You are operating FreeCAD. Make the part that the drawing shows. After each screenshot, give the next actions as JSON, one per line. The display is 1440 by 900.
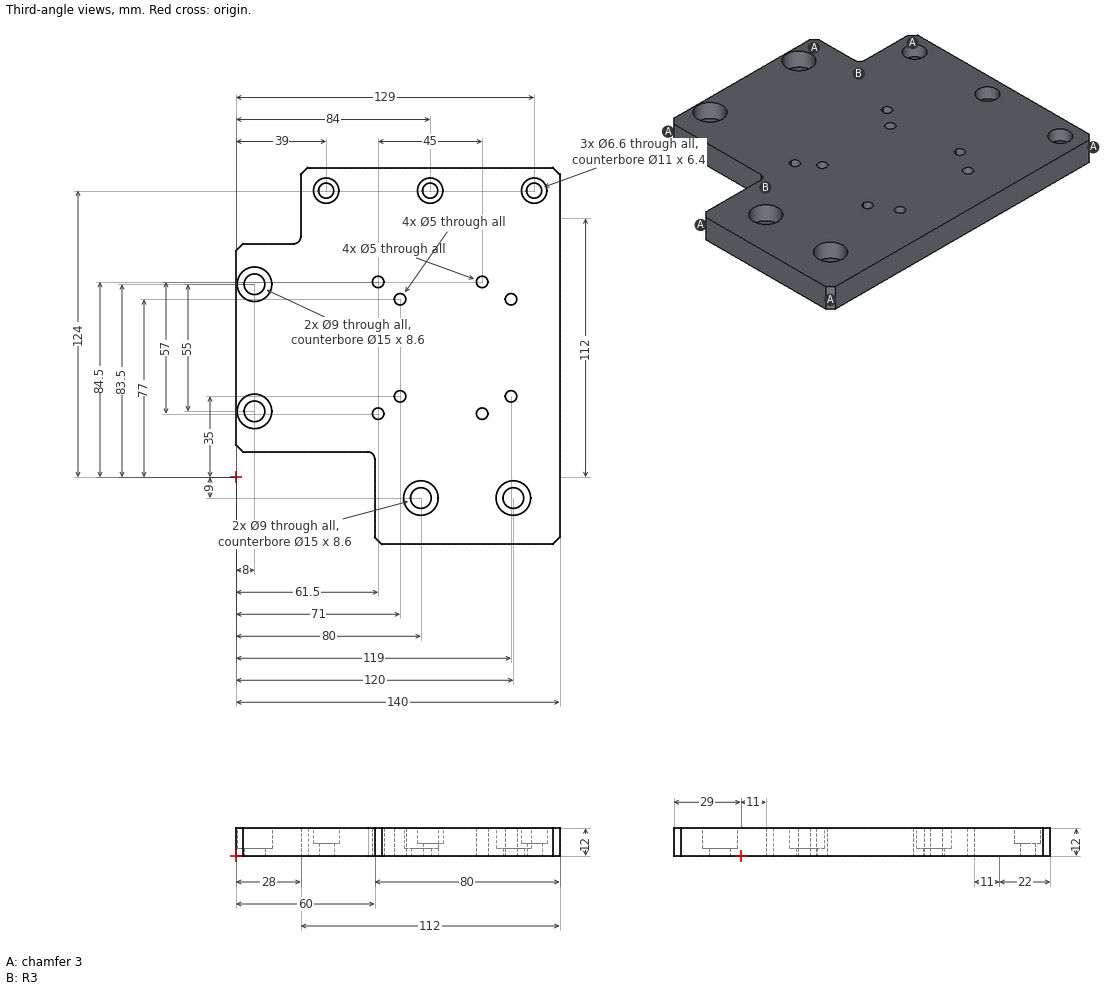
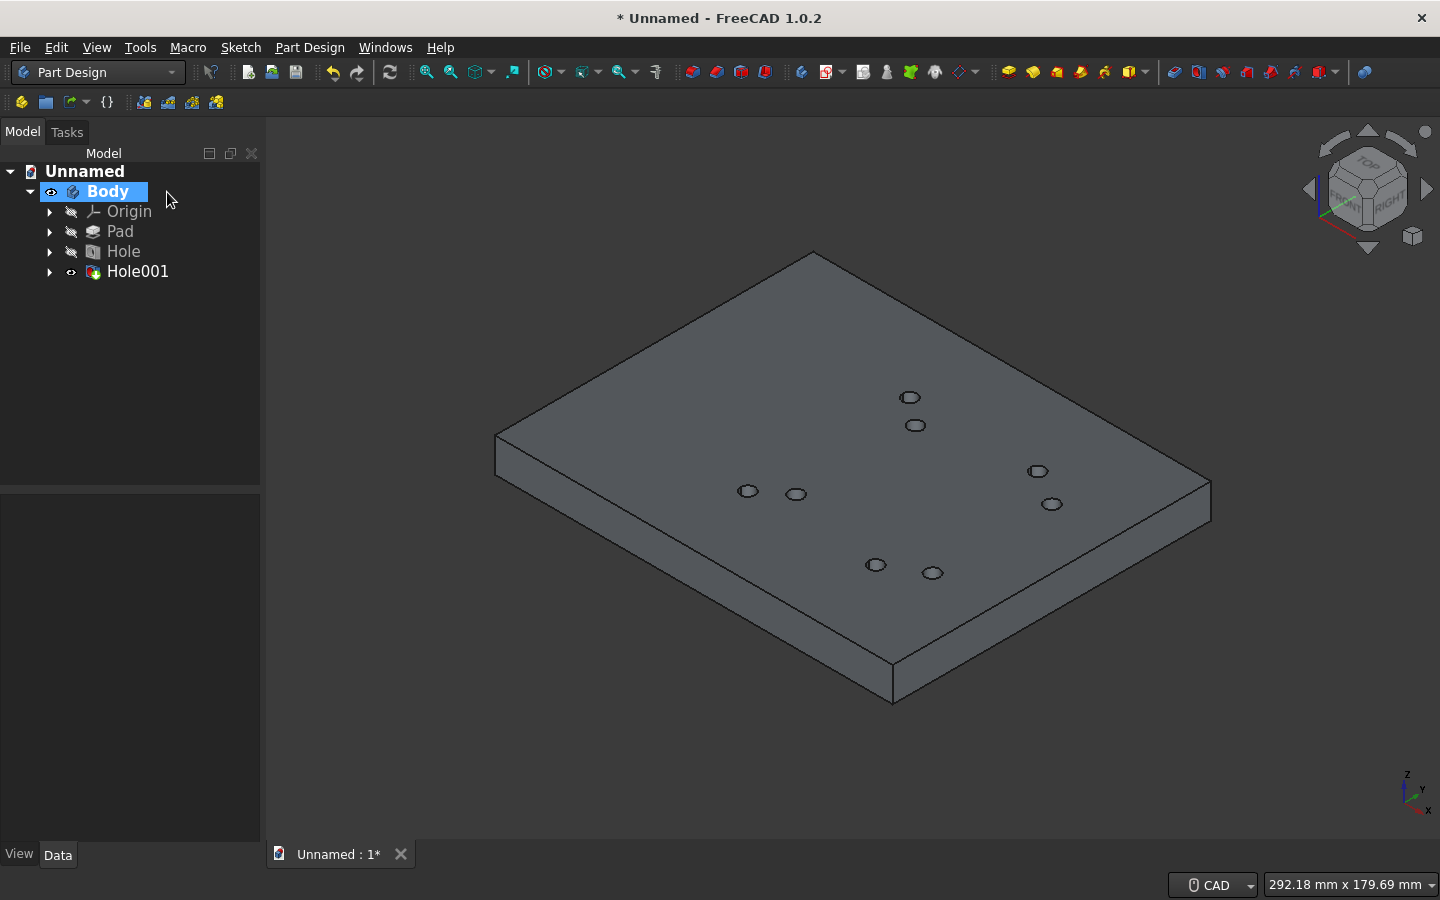
{"action": "key", "text": "4"}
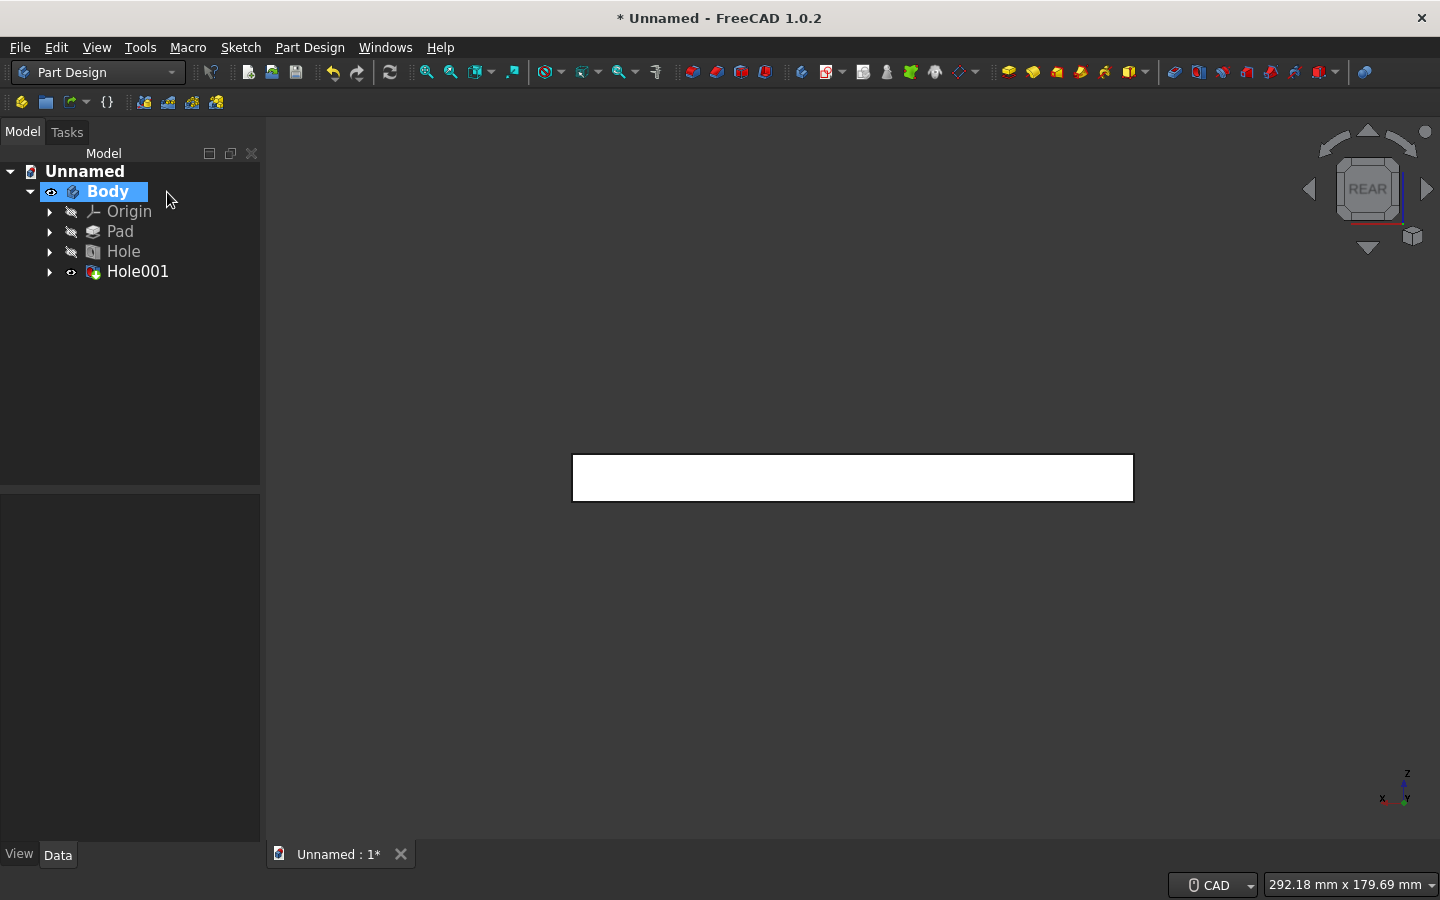
{"action": "left_click", "coordinate": [612, 477]}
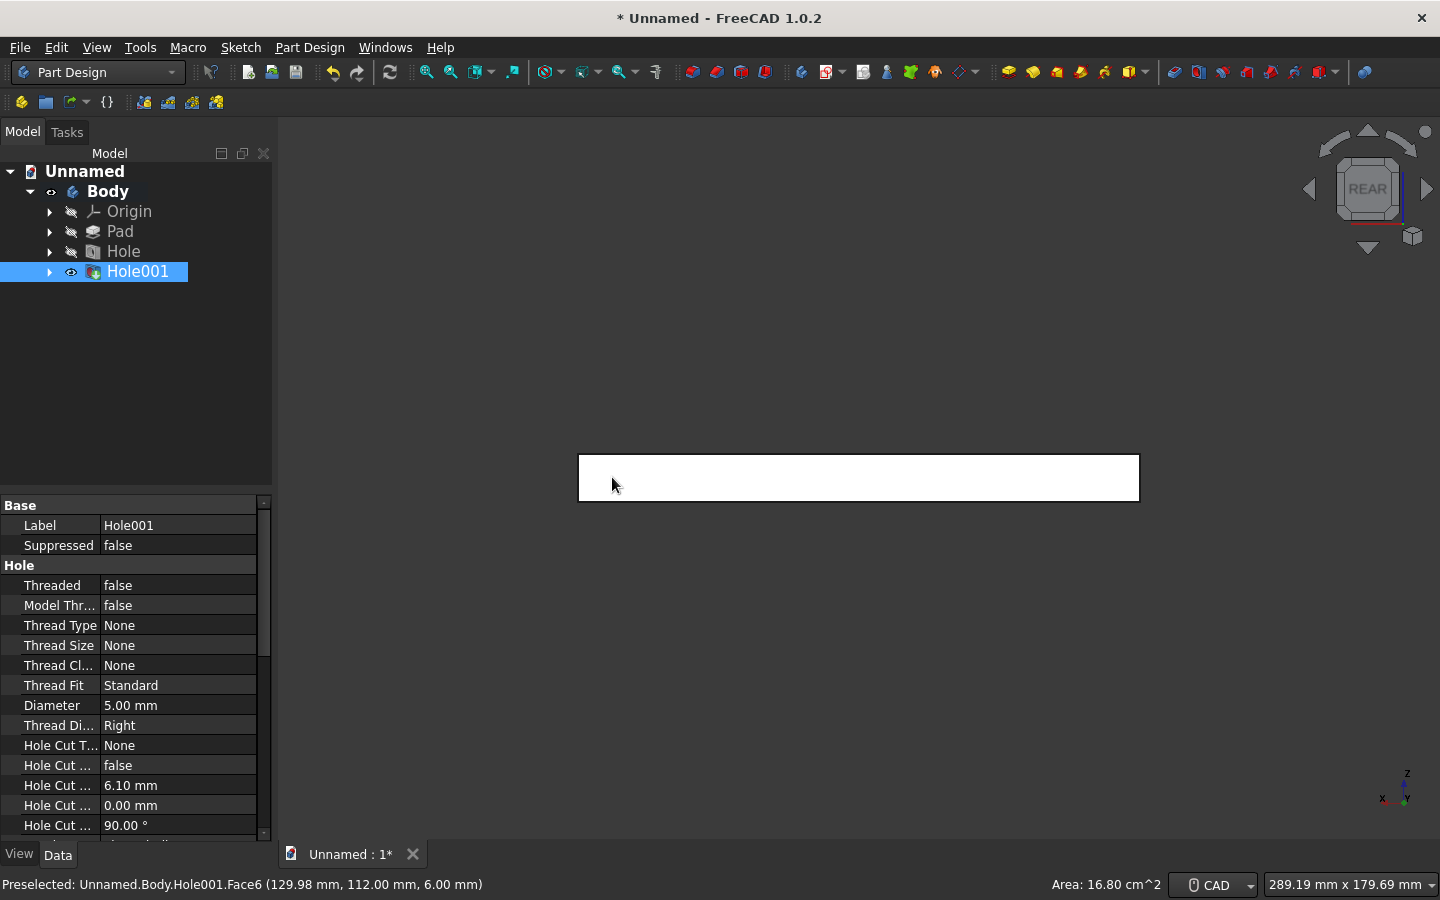
{"action": "left_click", "coordinate": [826, 72]}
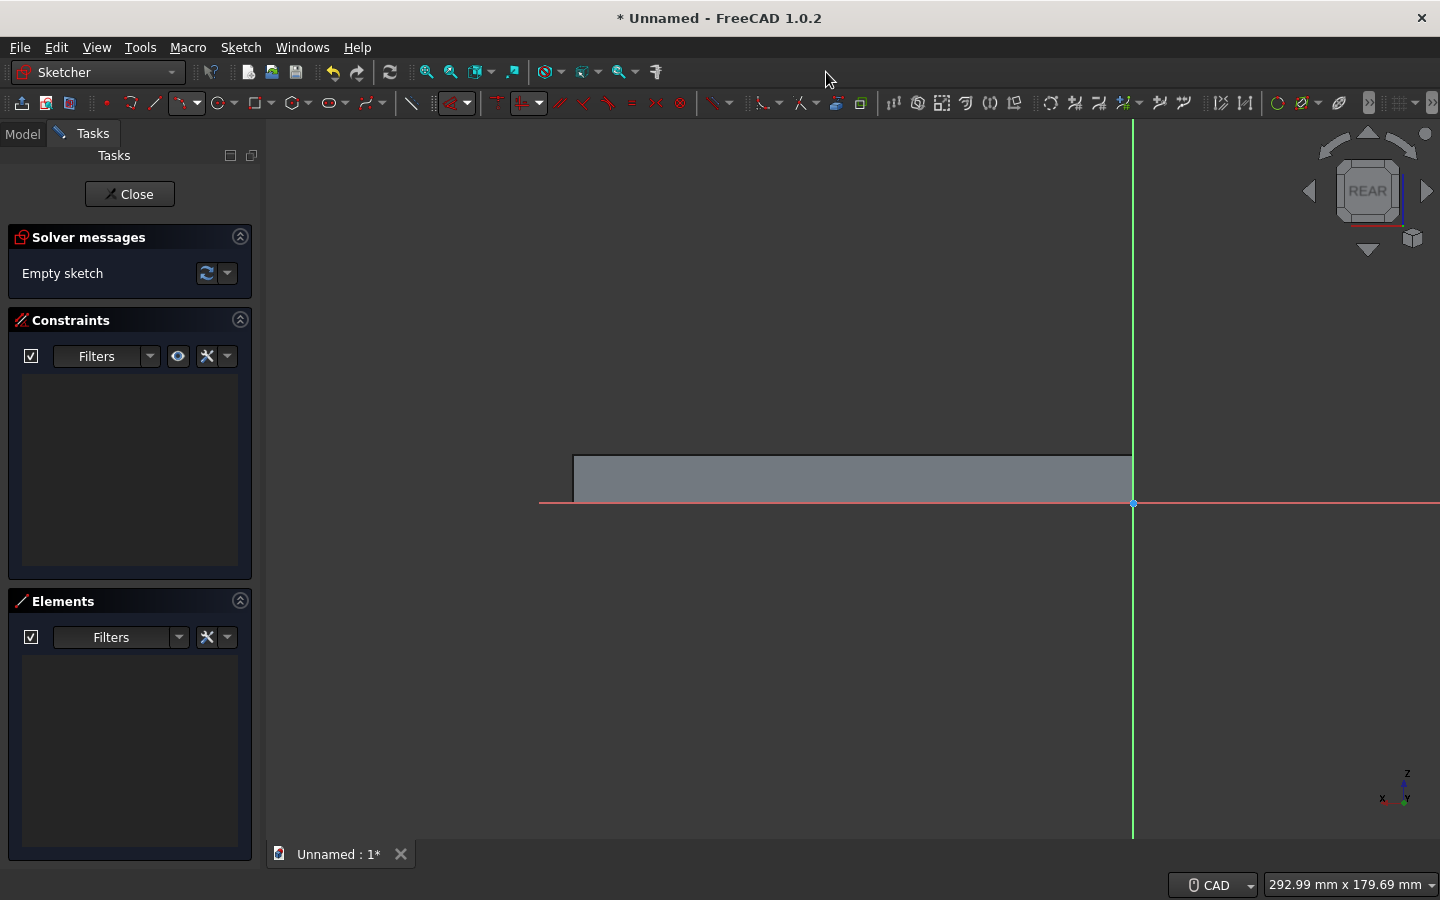
{"action": "key", "text": "g r"}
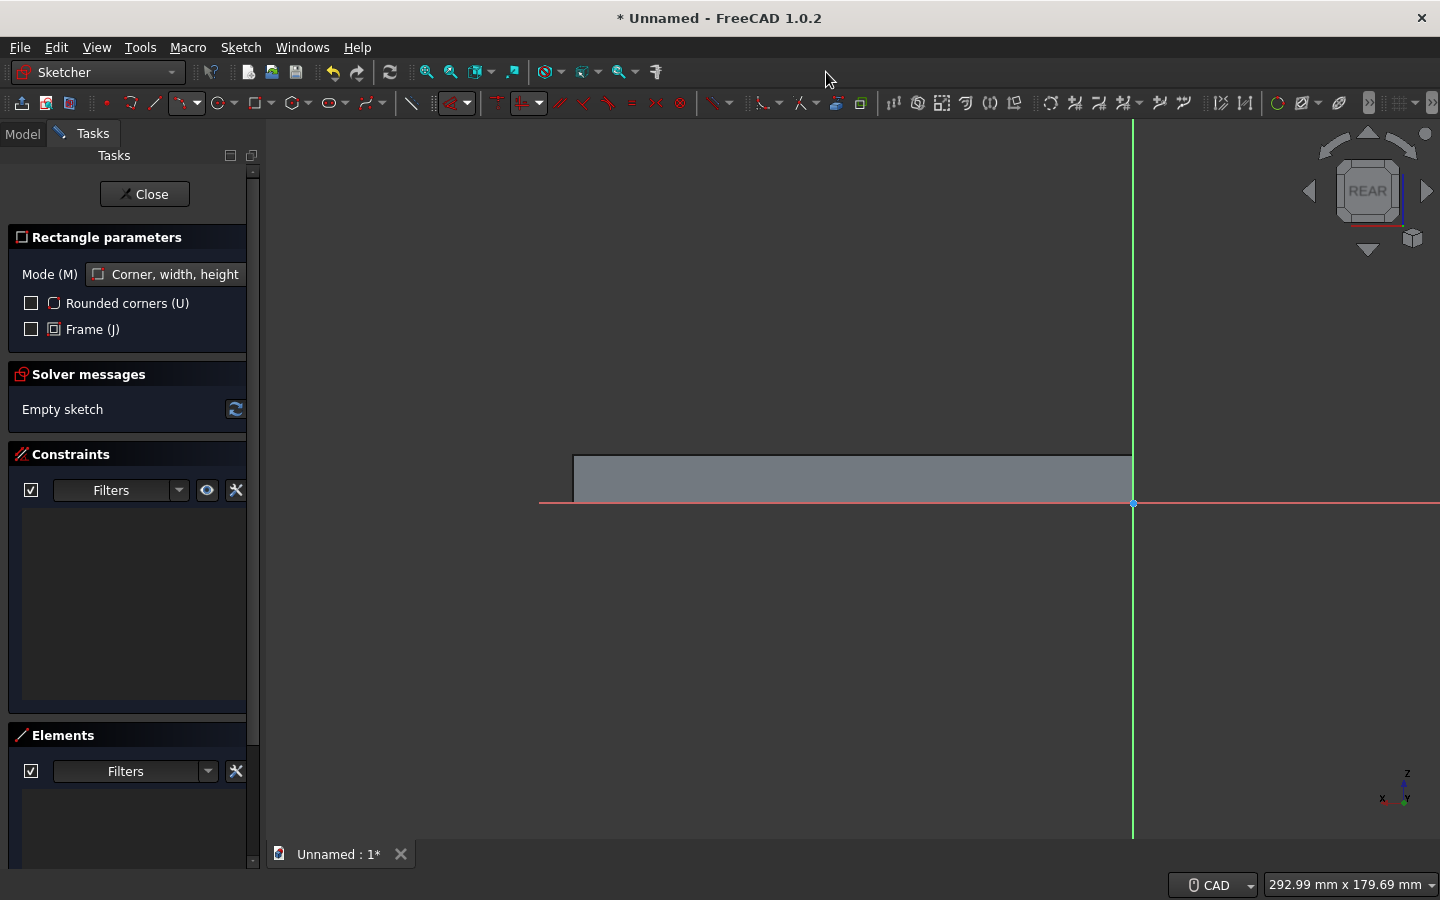
{"action": "left_click", "coordinate": [573, 455]}
{"action": "left_click", "coordinate": [1021, 503]}
{"action": "key", "text": "Escape"}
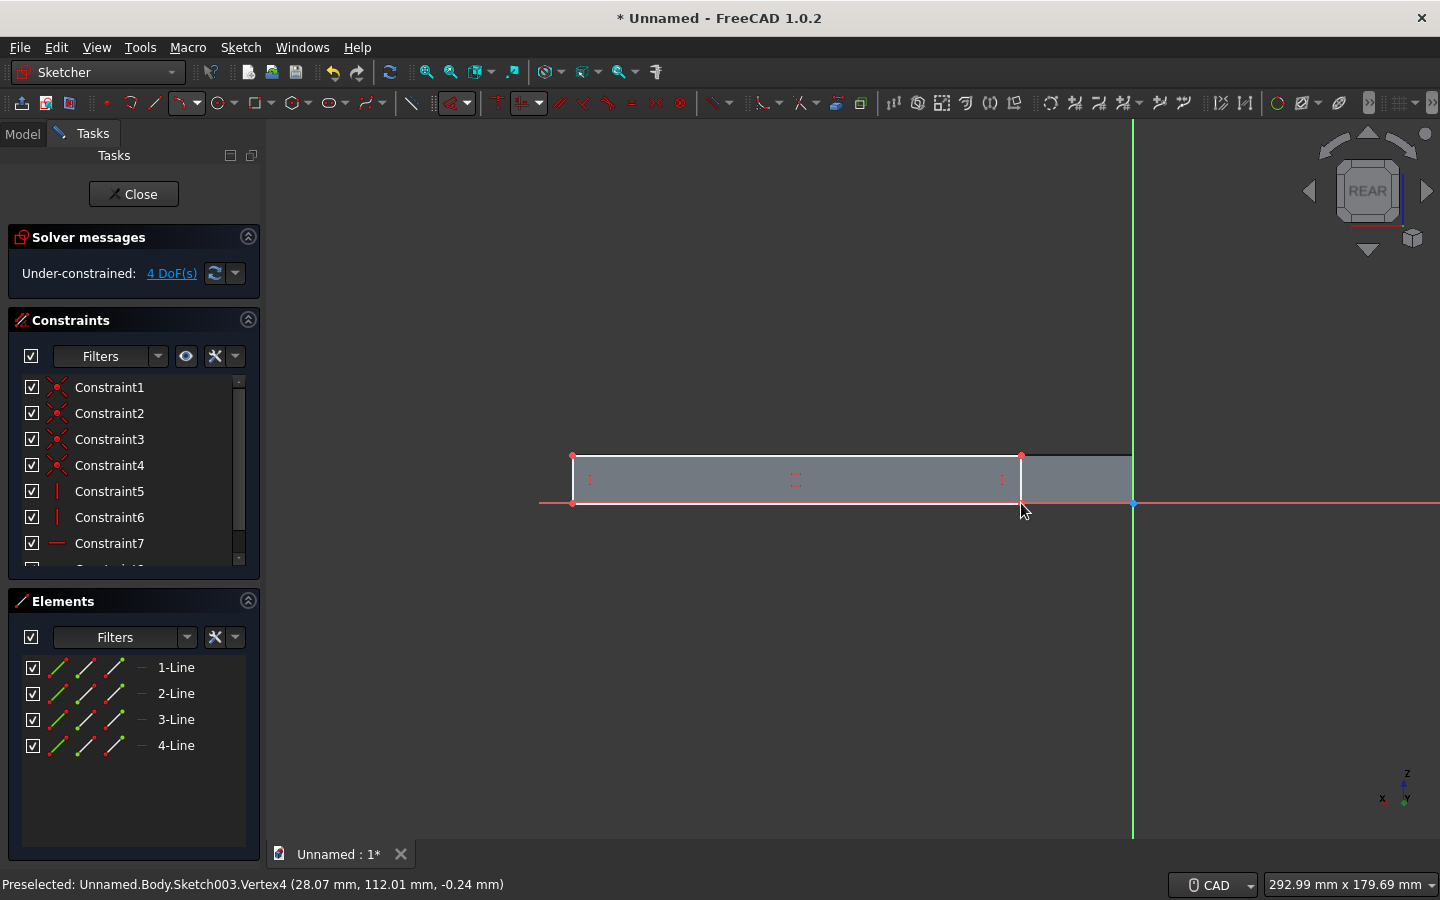
{"action": "left_click", "coordinate": [573, 504]}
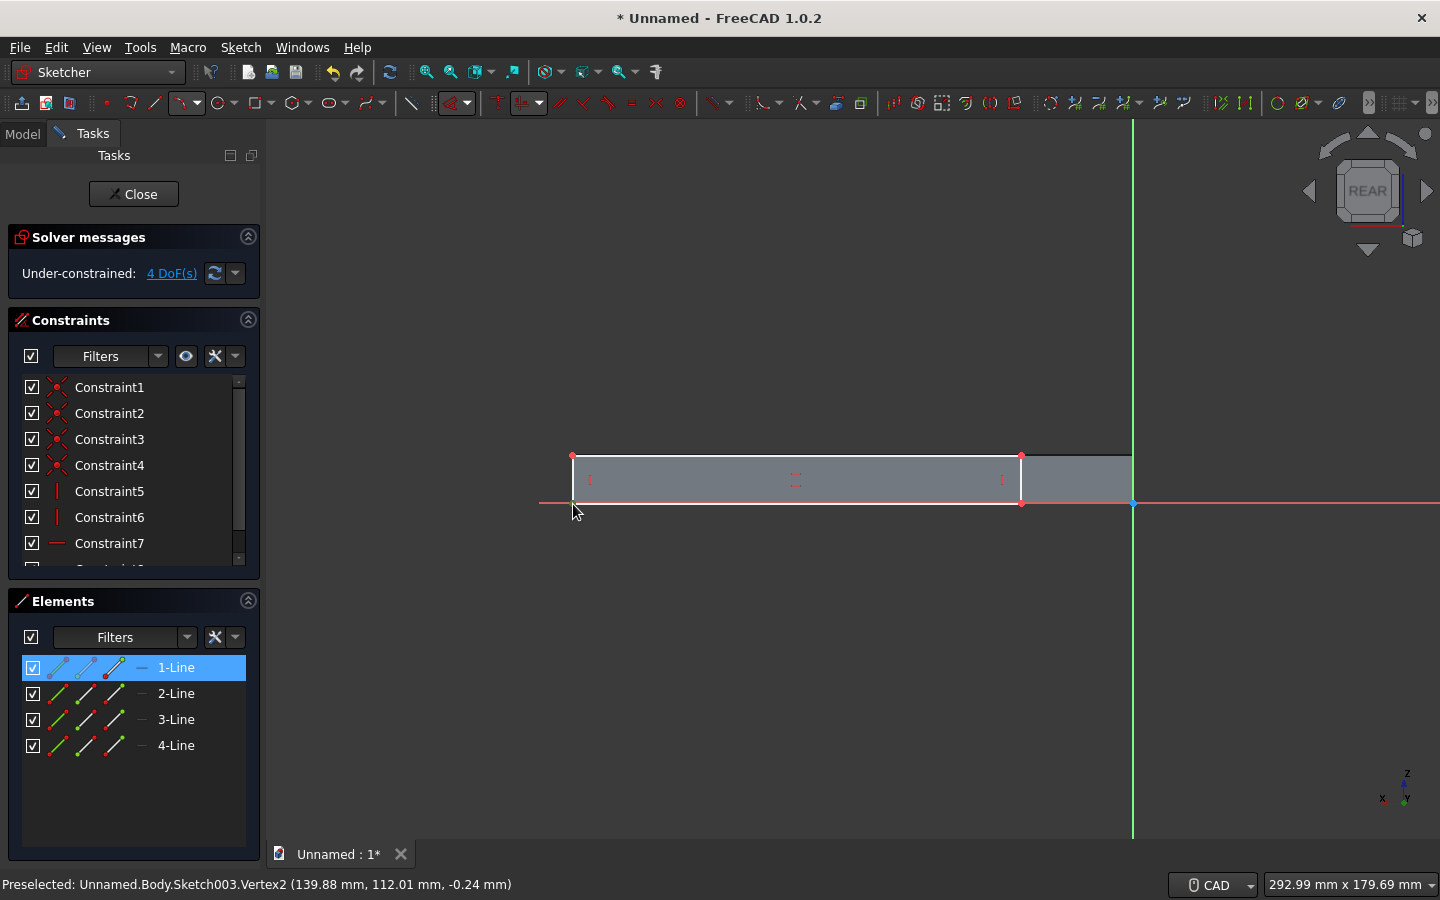
{"action": "left_click", "coordinate": [1065, 503]}